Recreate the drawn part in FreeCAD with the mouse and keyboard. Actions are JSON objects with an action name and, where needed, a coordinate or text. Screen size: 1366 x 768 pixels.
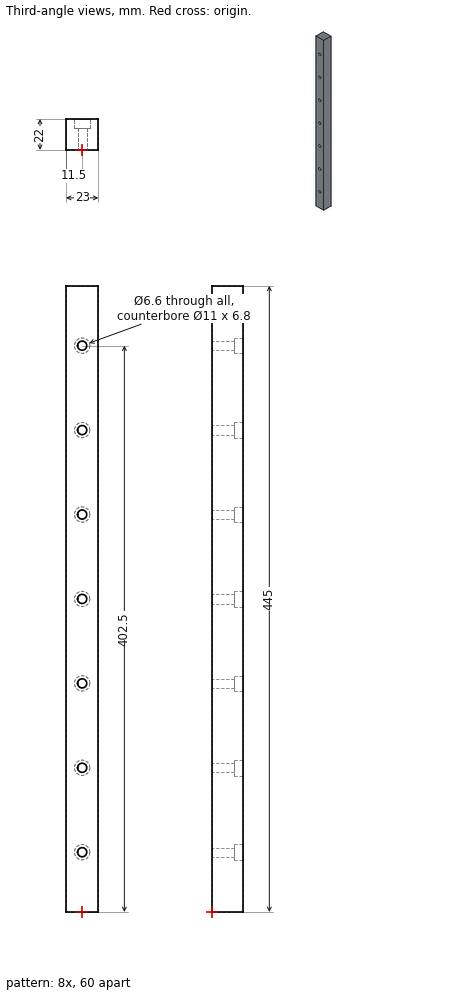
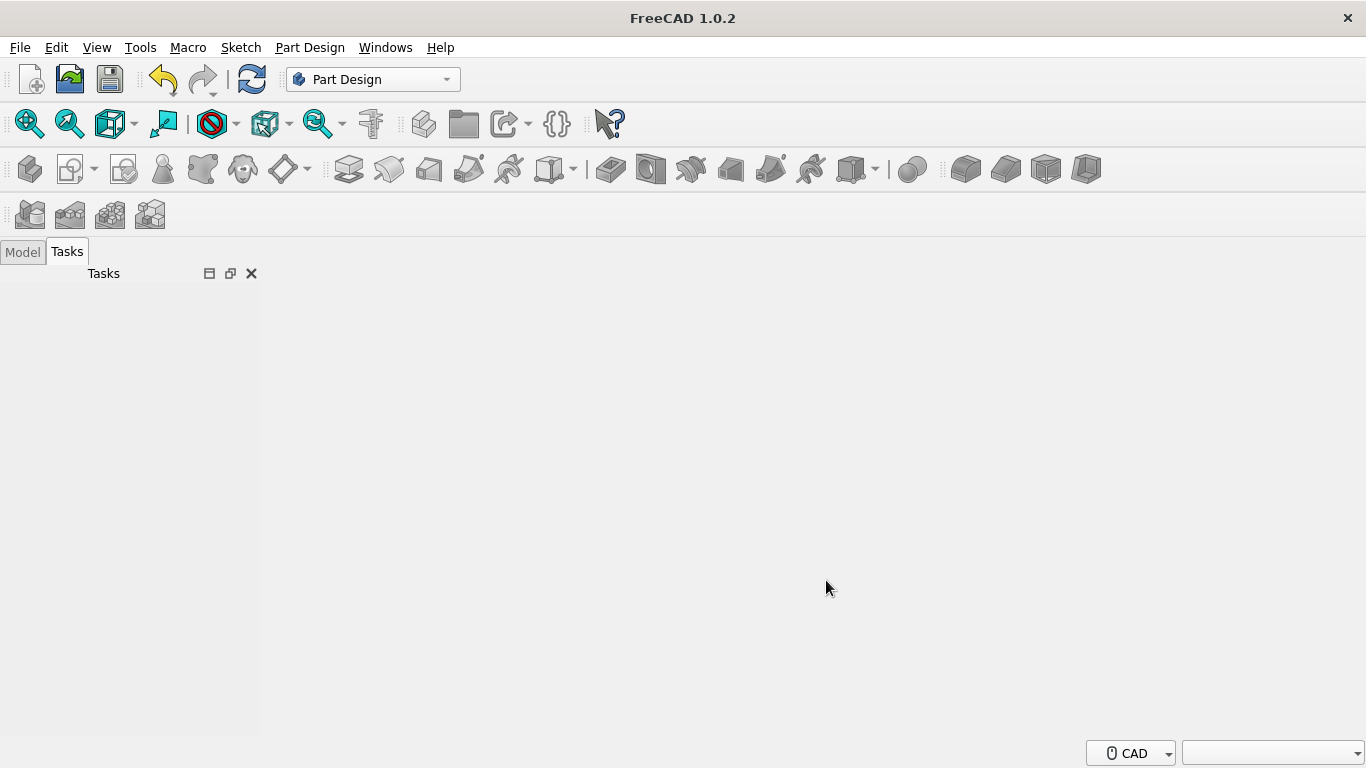
{"action": "left_click", "coordinate": [30, 80]}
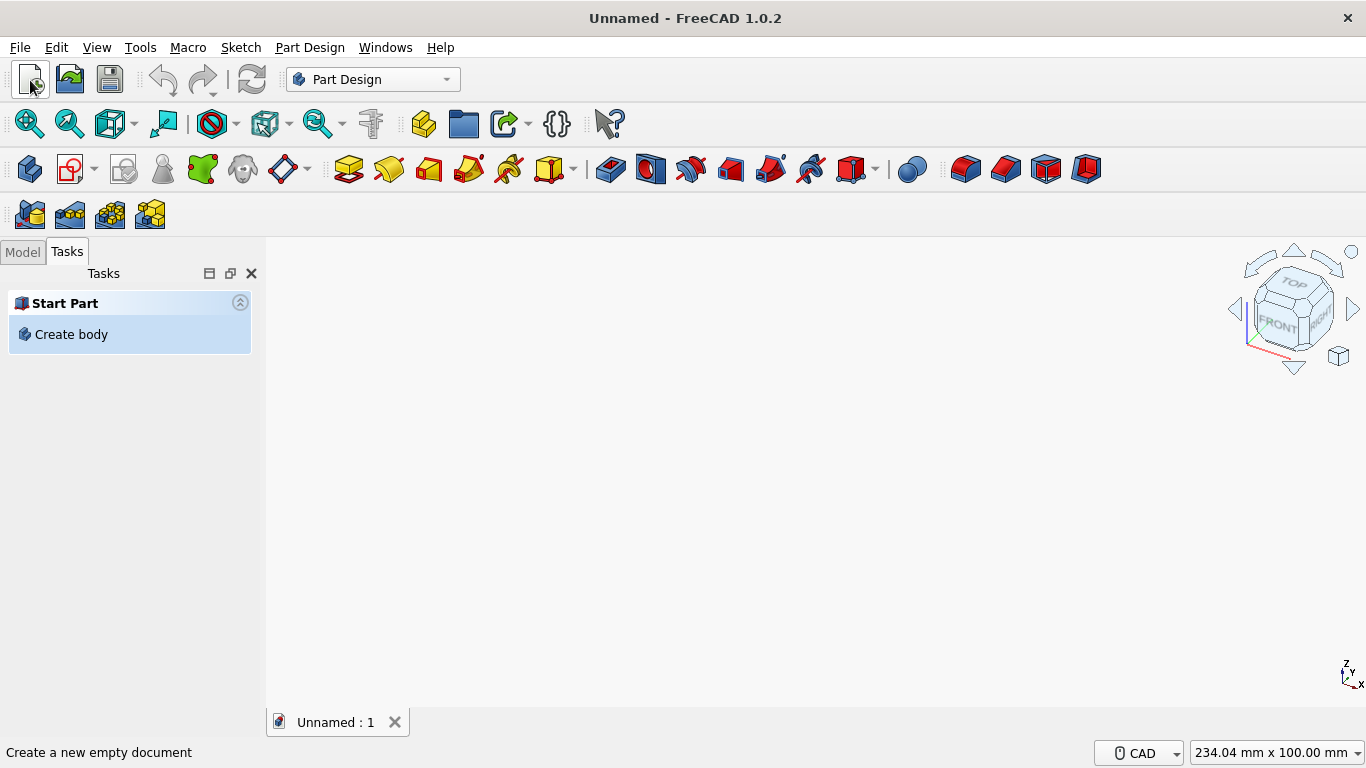
{"action": "left_click", "coordinate": [70, 170]}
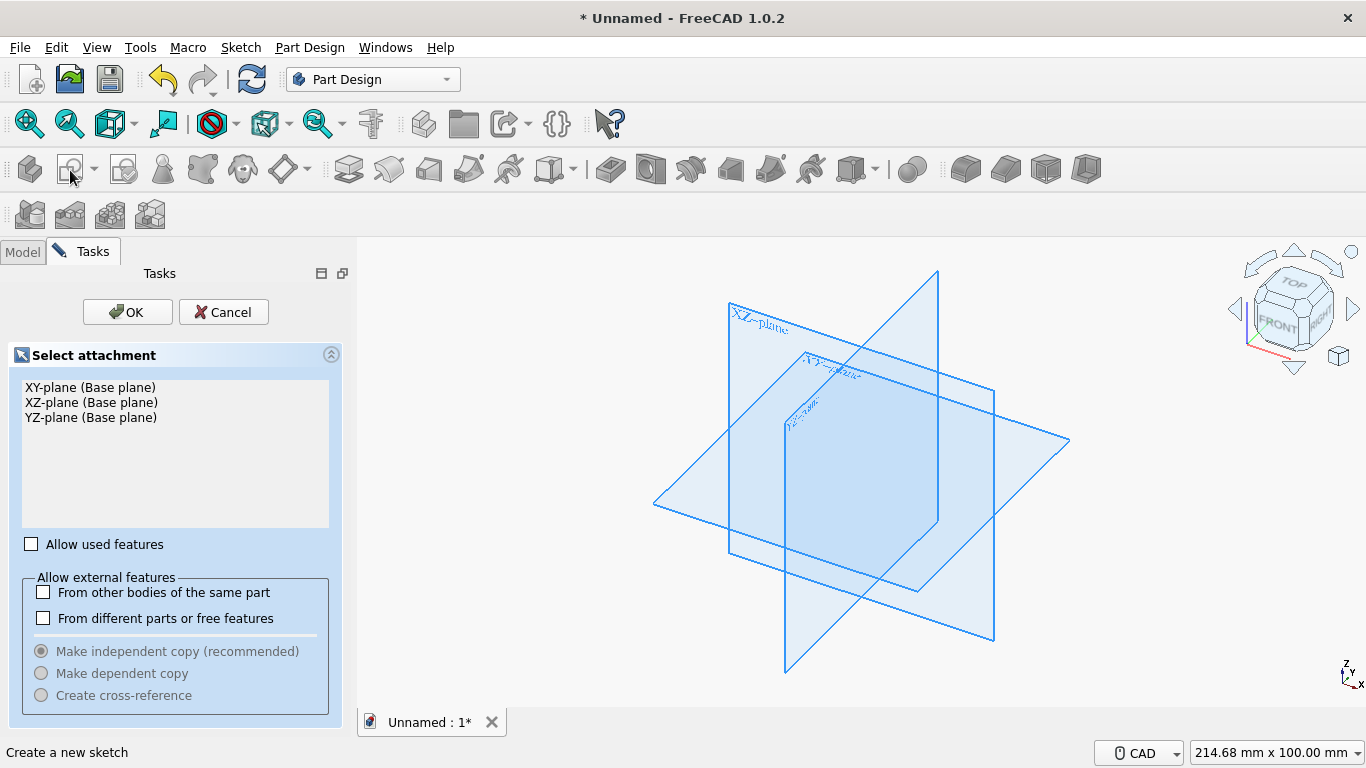
{"action": "left_click", "coordinate": [82, 388]}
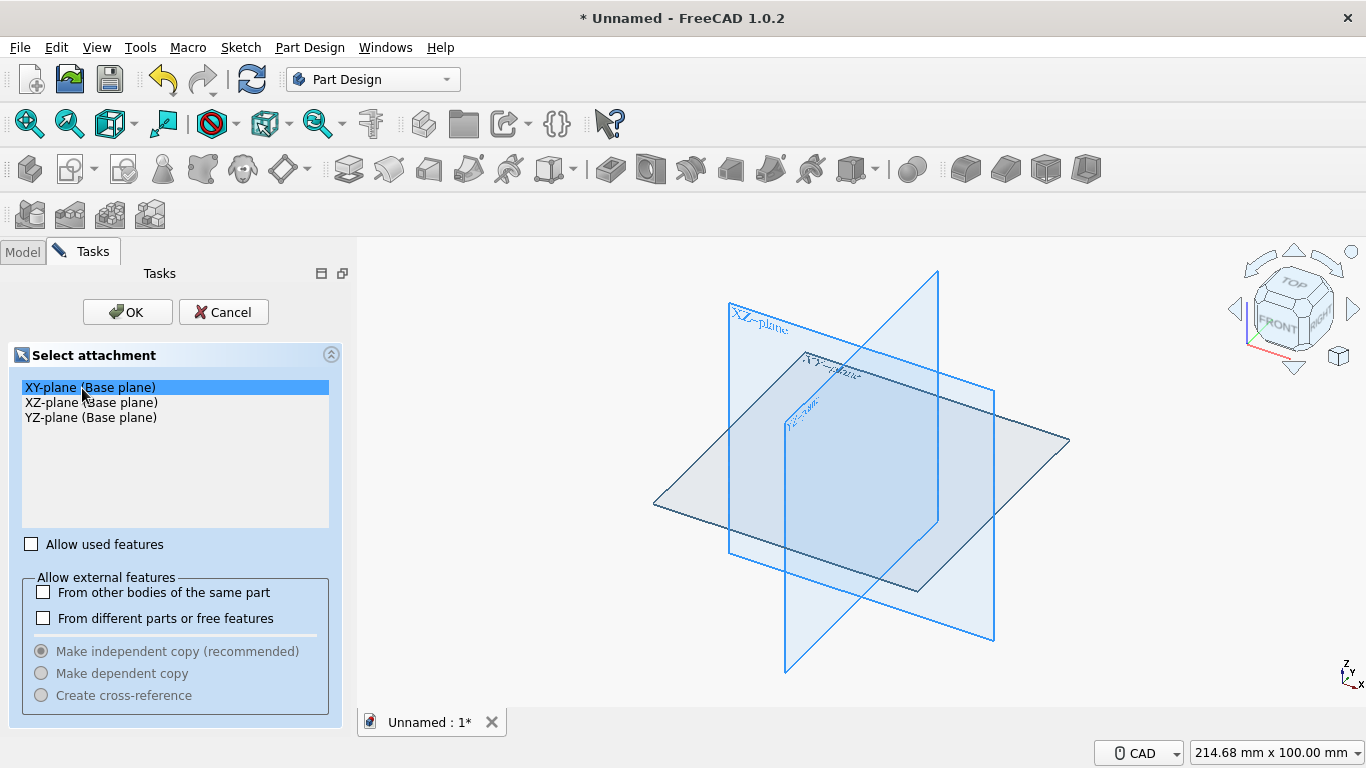
{"action": "left_click", "coordinate": [128, 312]}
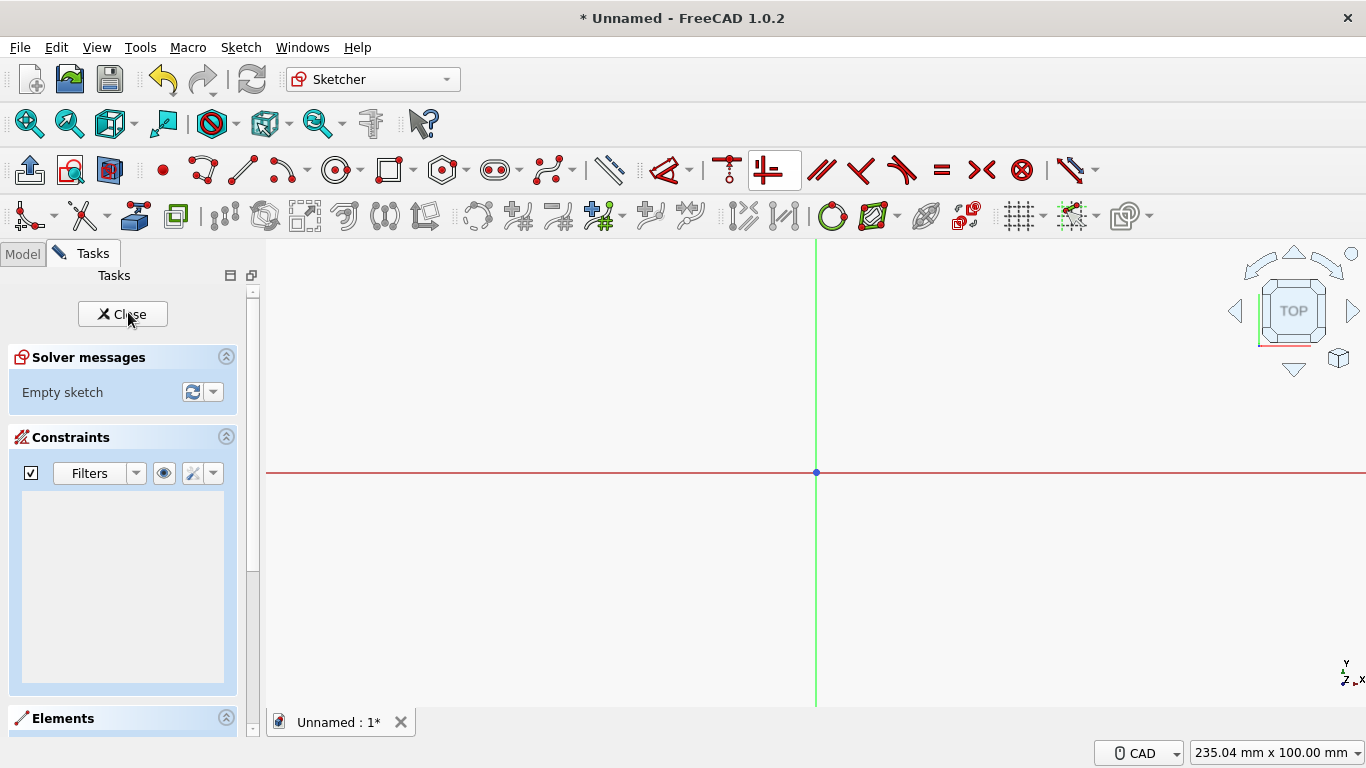
{"action": "scroll", "coordinate": [856, 392], "scroll_direction": "up", "scroll_amount": 5}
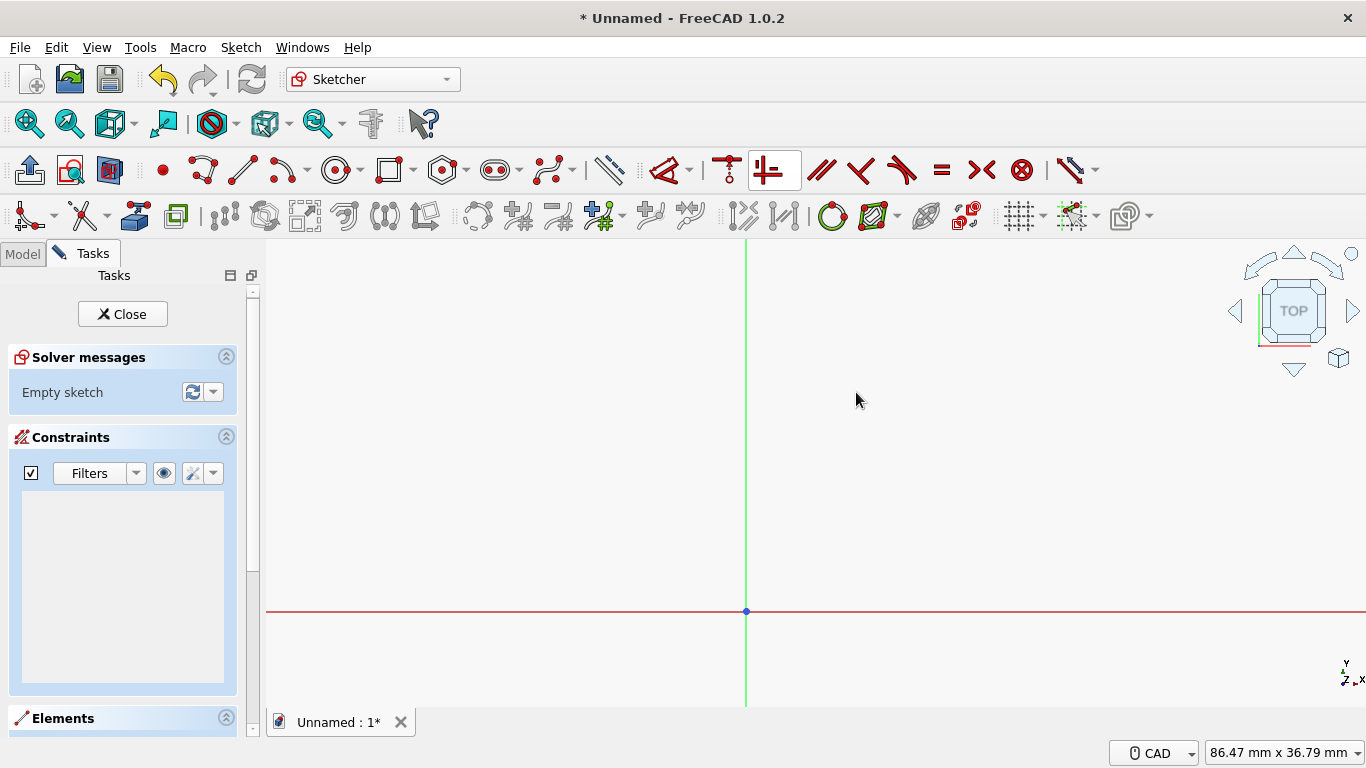
{"action": "left_click", "coordinate": [390, 170]}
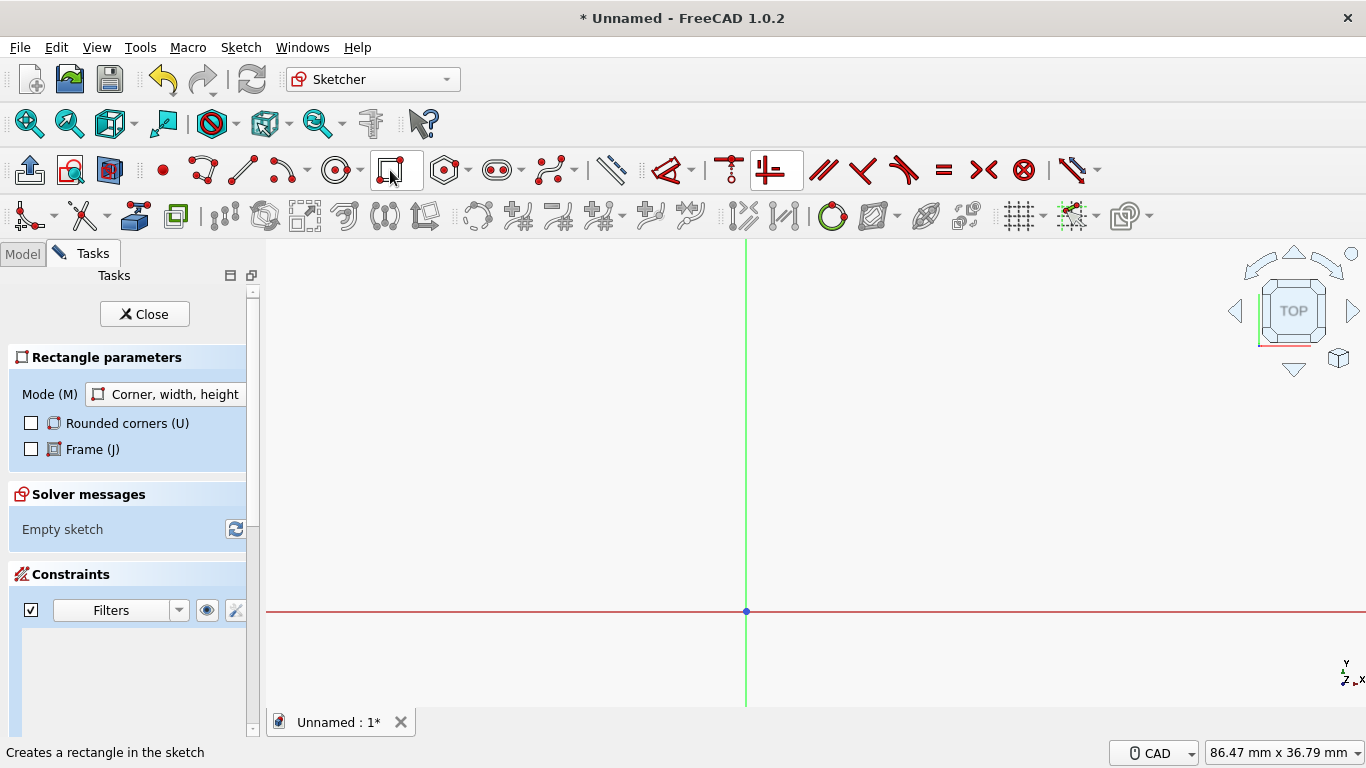
{"action": "left_click", "coordinate": [600, 332]}
{"action": "left_click", "coordinate": [893, 612]}
{"action": "key", "text": "Escape"}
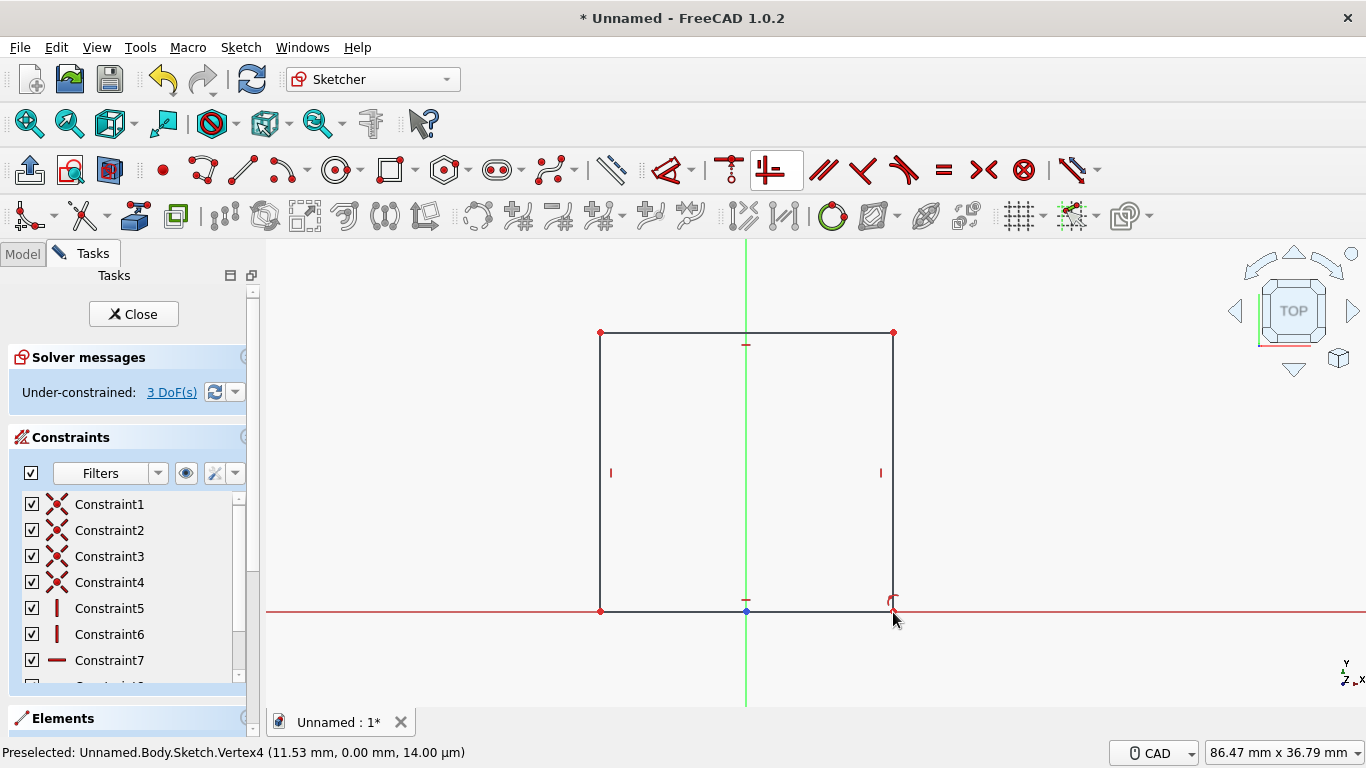
{"action": "key", "text": "d"}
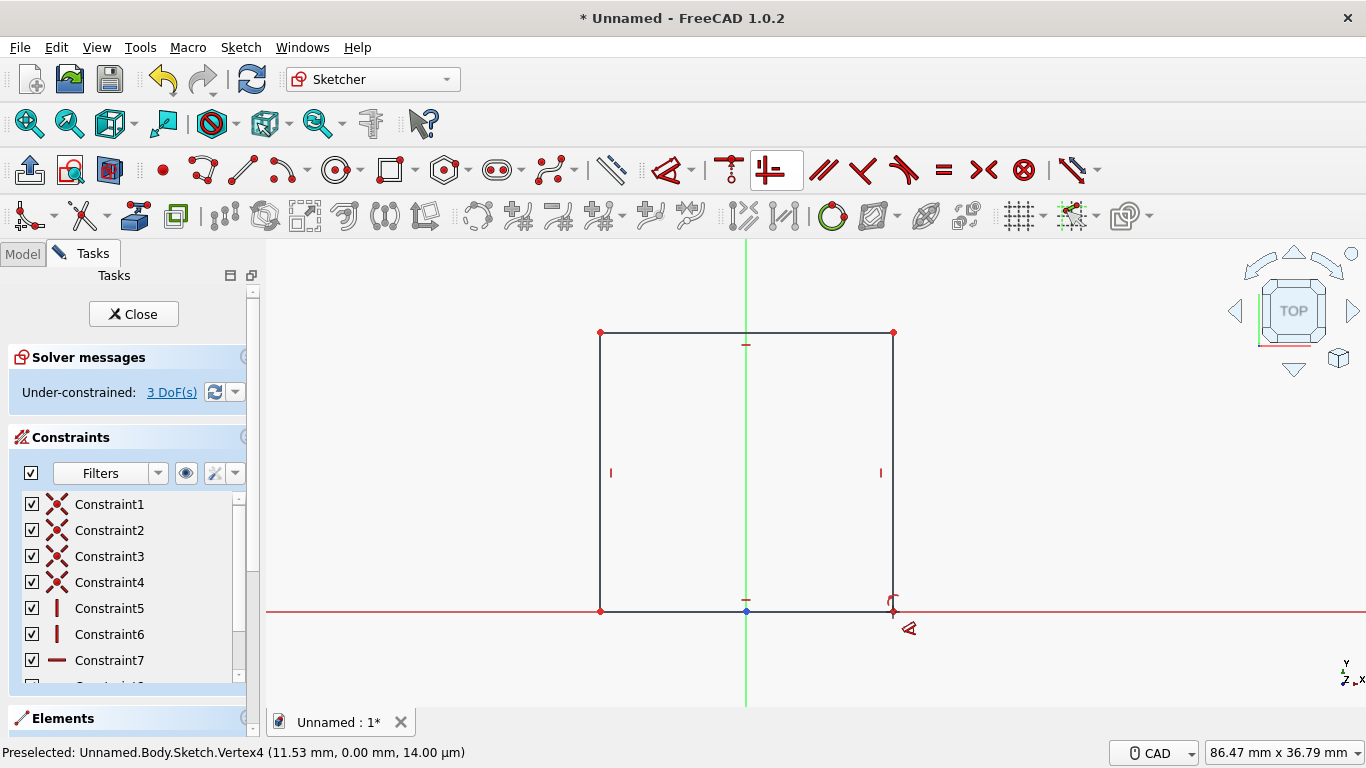
{"action": "left_click", "coordinate": [600, 417]}
{"action": "left_click", "coordinate": [566, 472]}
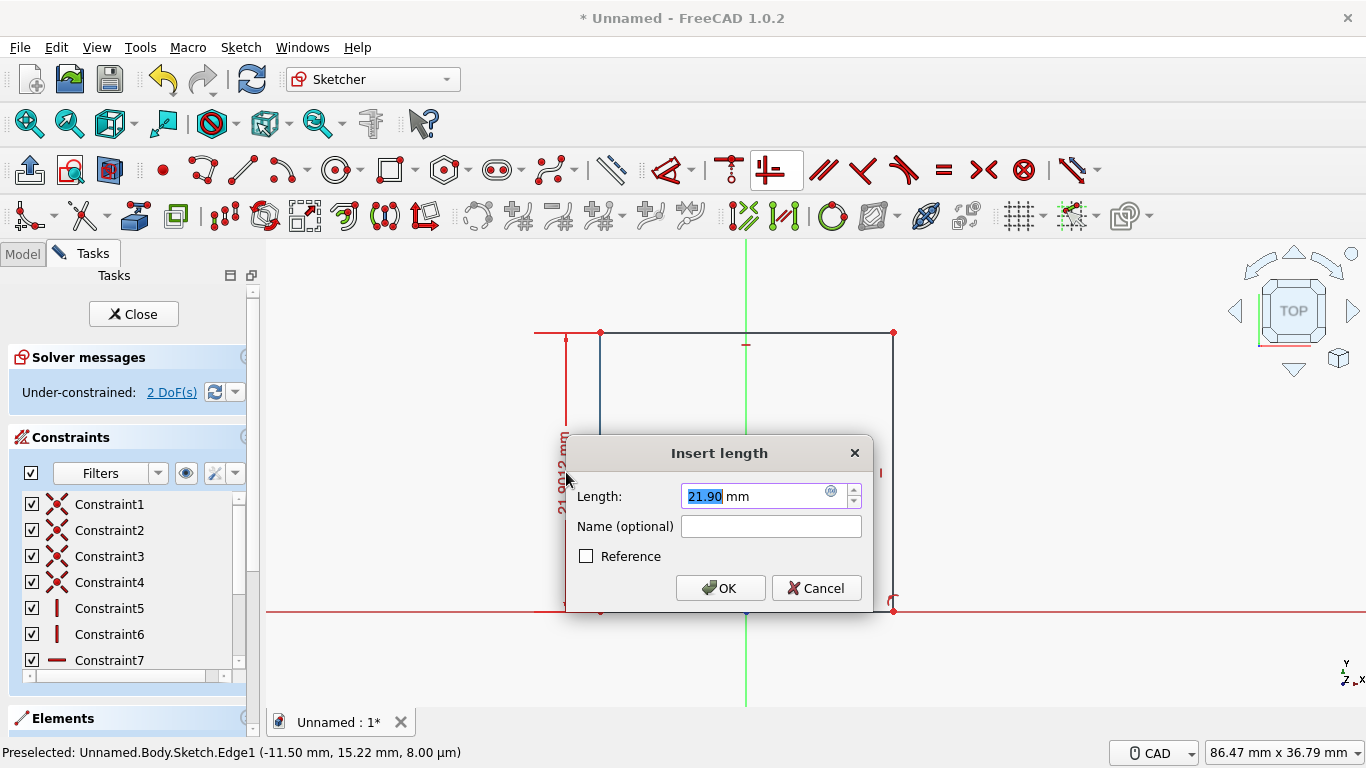
{"action": "type", "text": "22"}
{"action": "key", "text": "Return"}